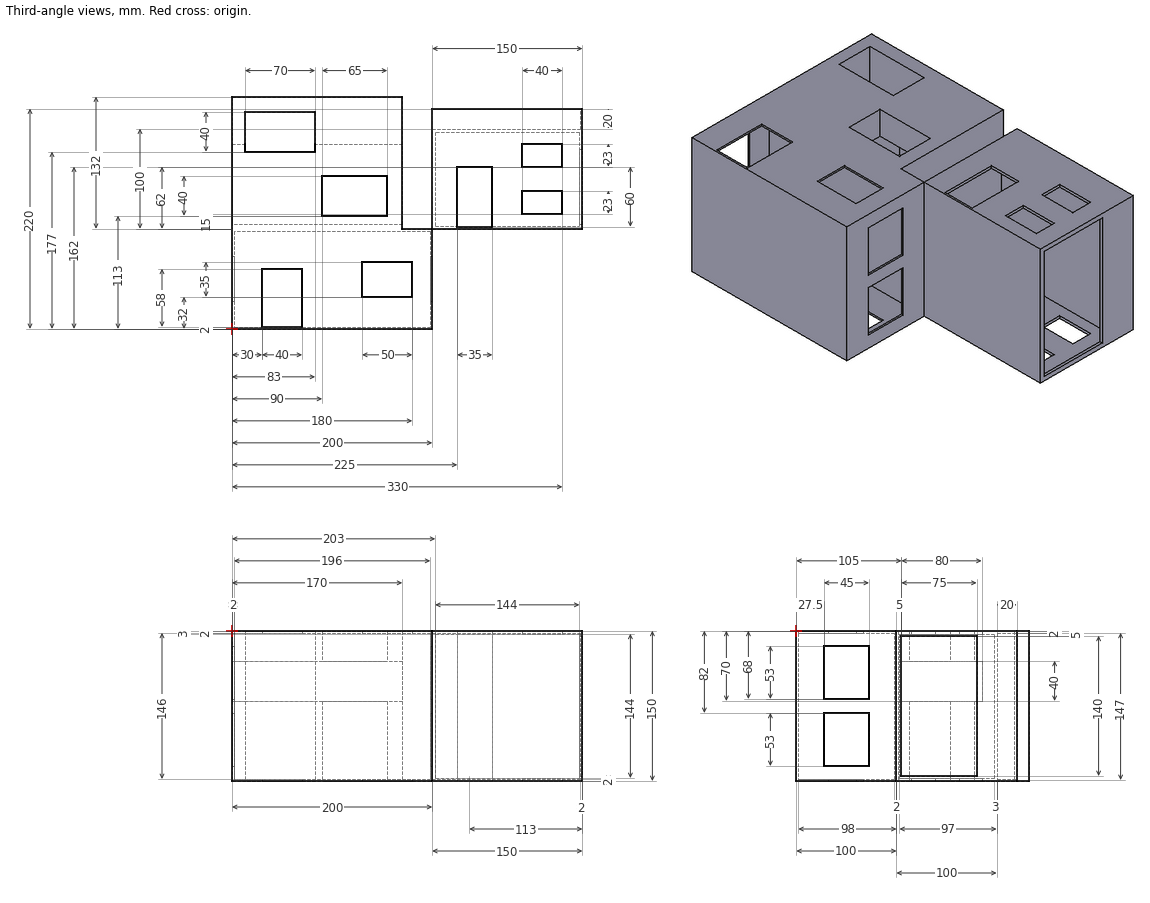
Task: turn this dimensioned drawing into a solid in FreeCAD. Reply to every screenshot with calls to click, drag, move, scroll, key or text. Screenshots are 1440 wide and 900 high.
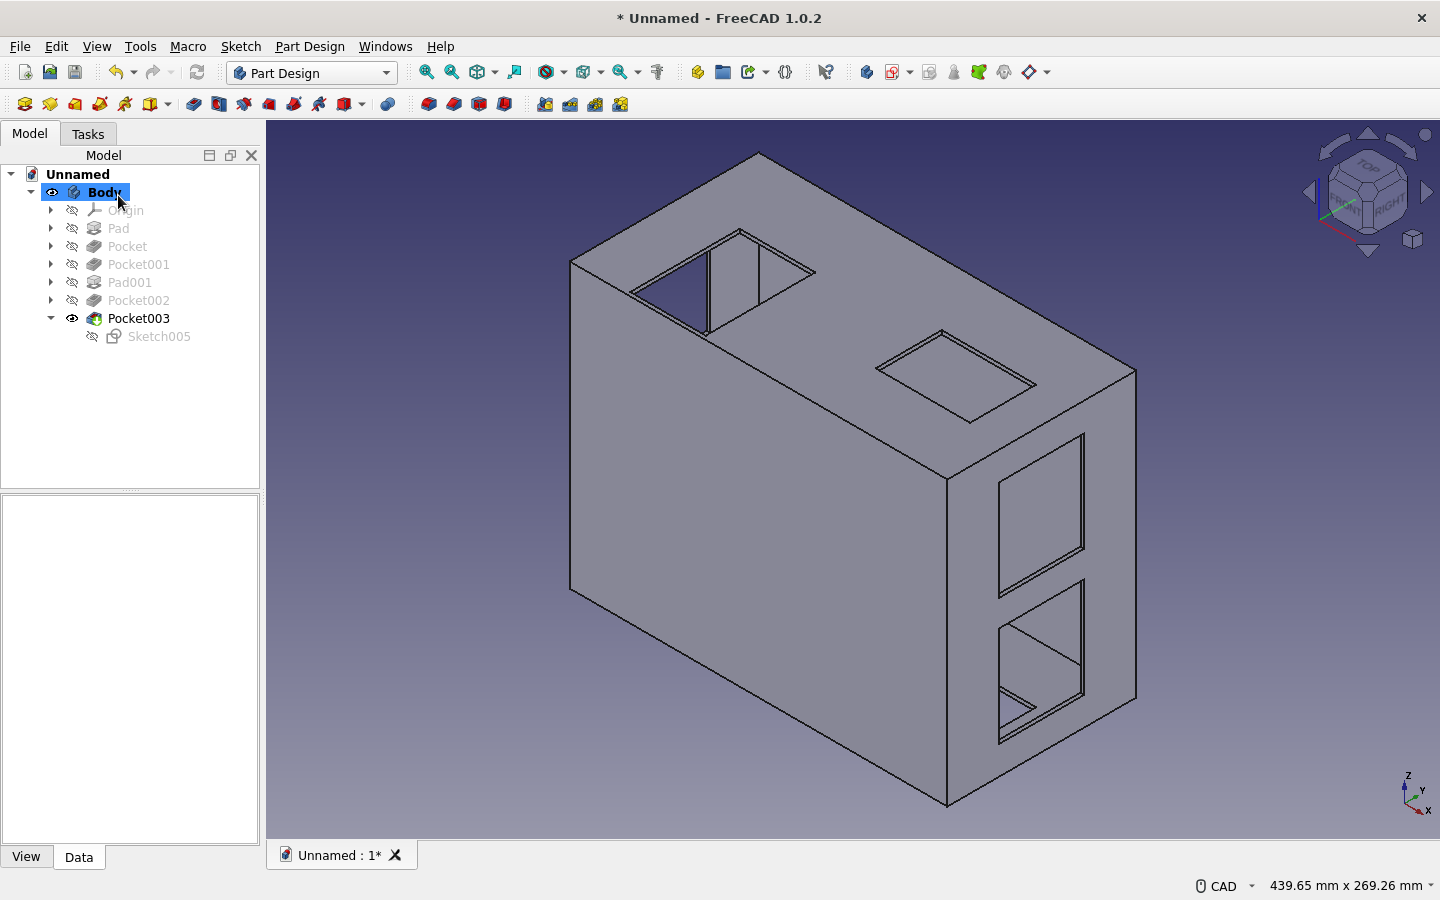
key(4)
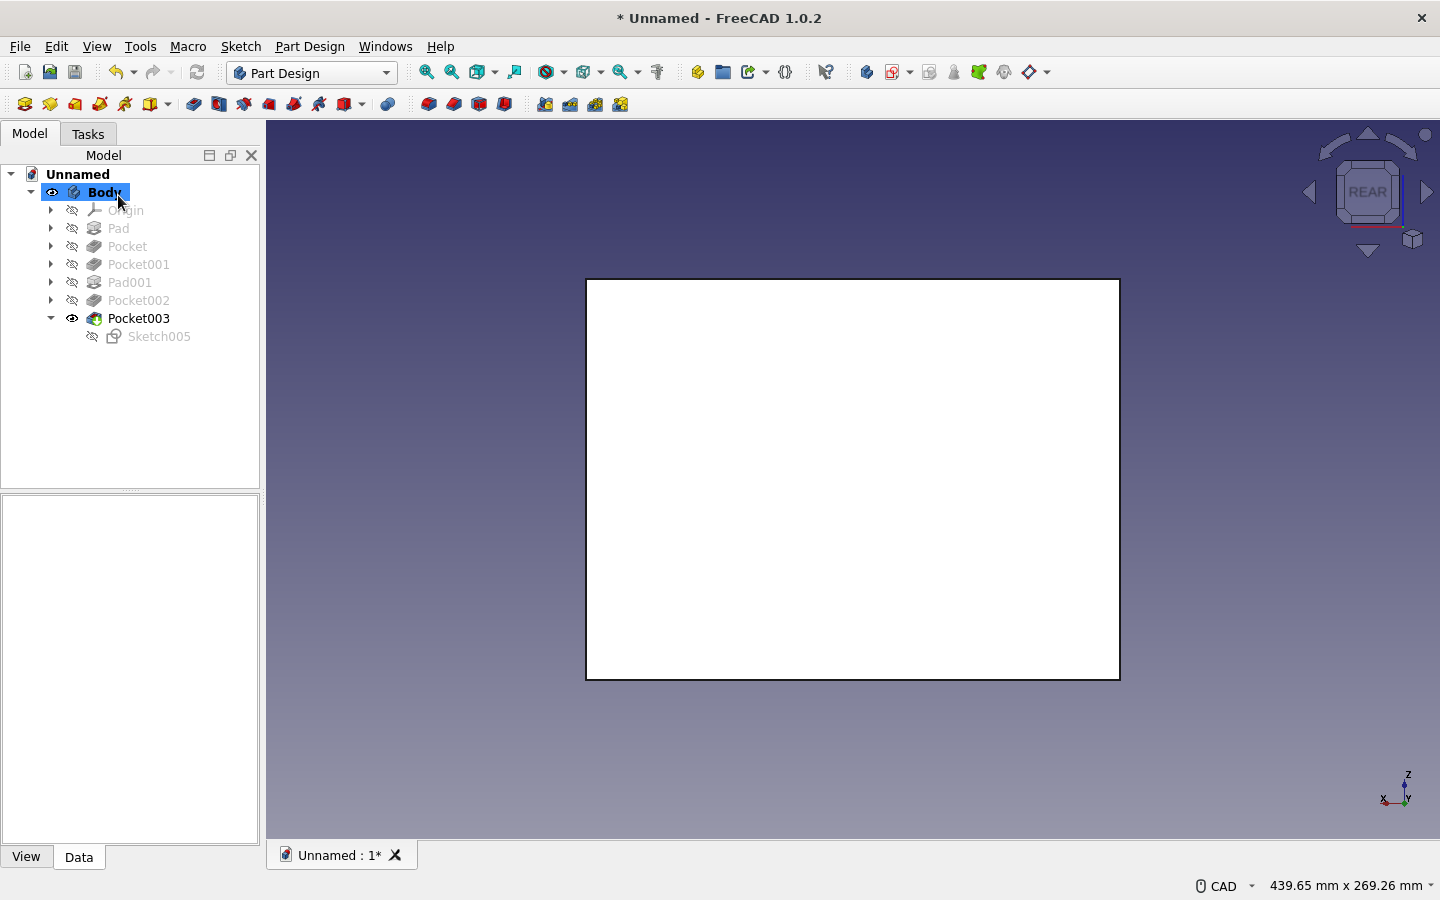
click(853, 478)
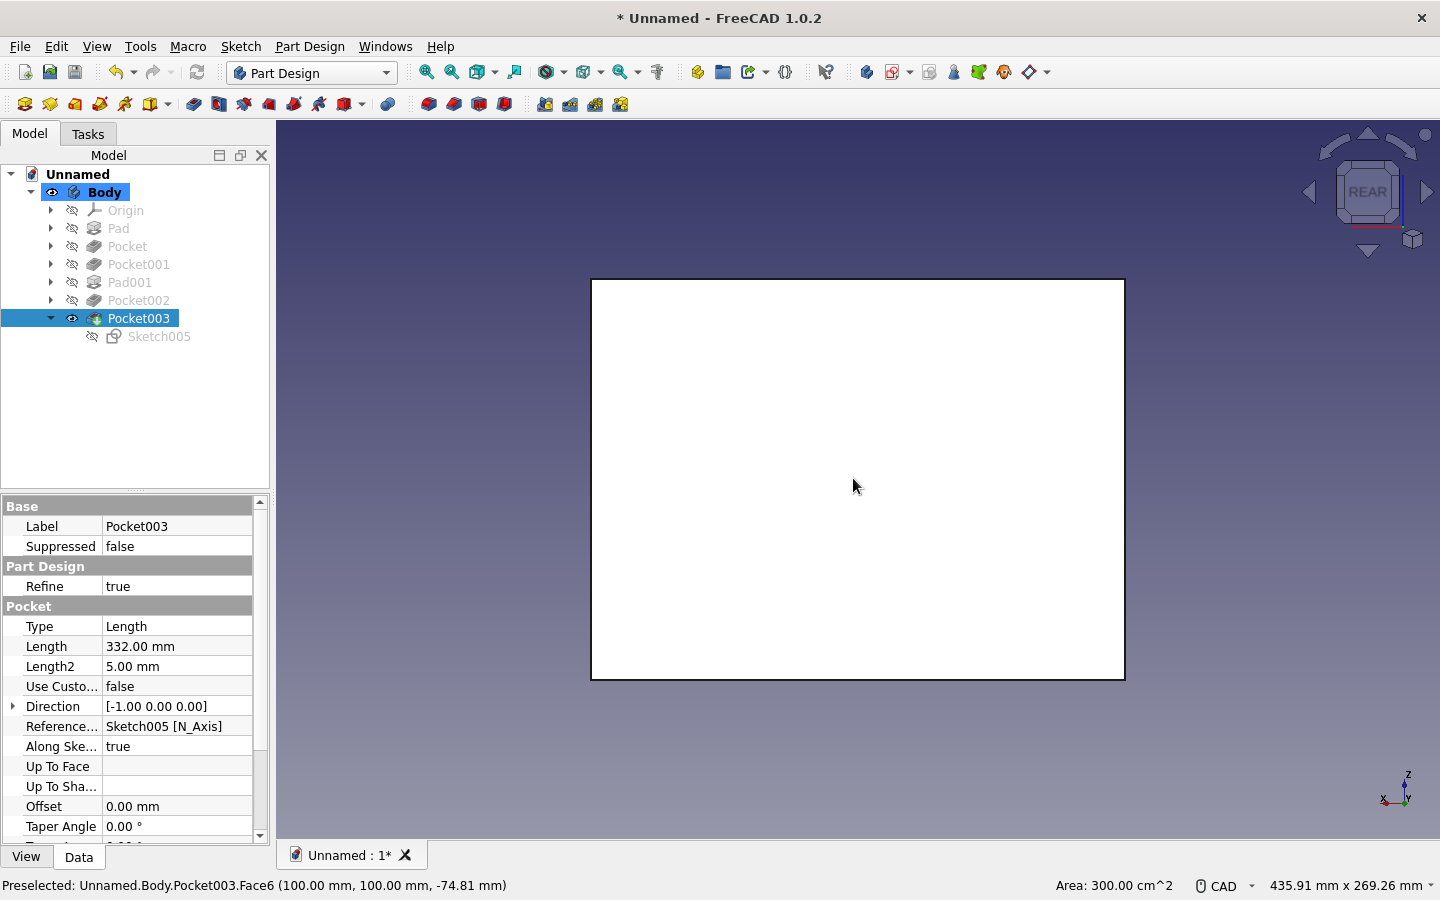
click(892, 72)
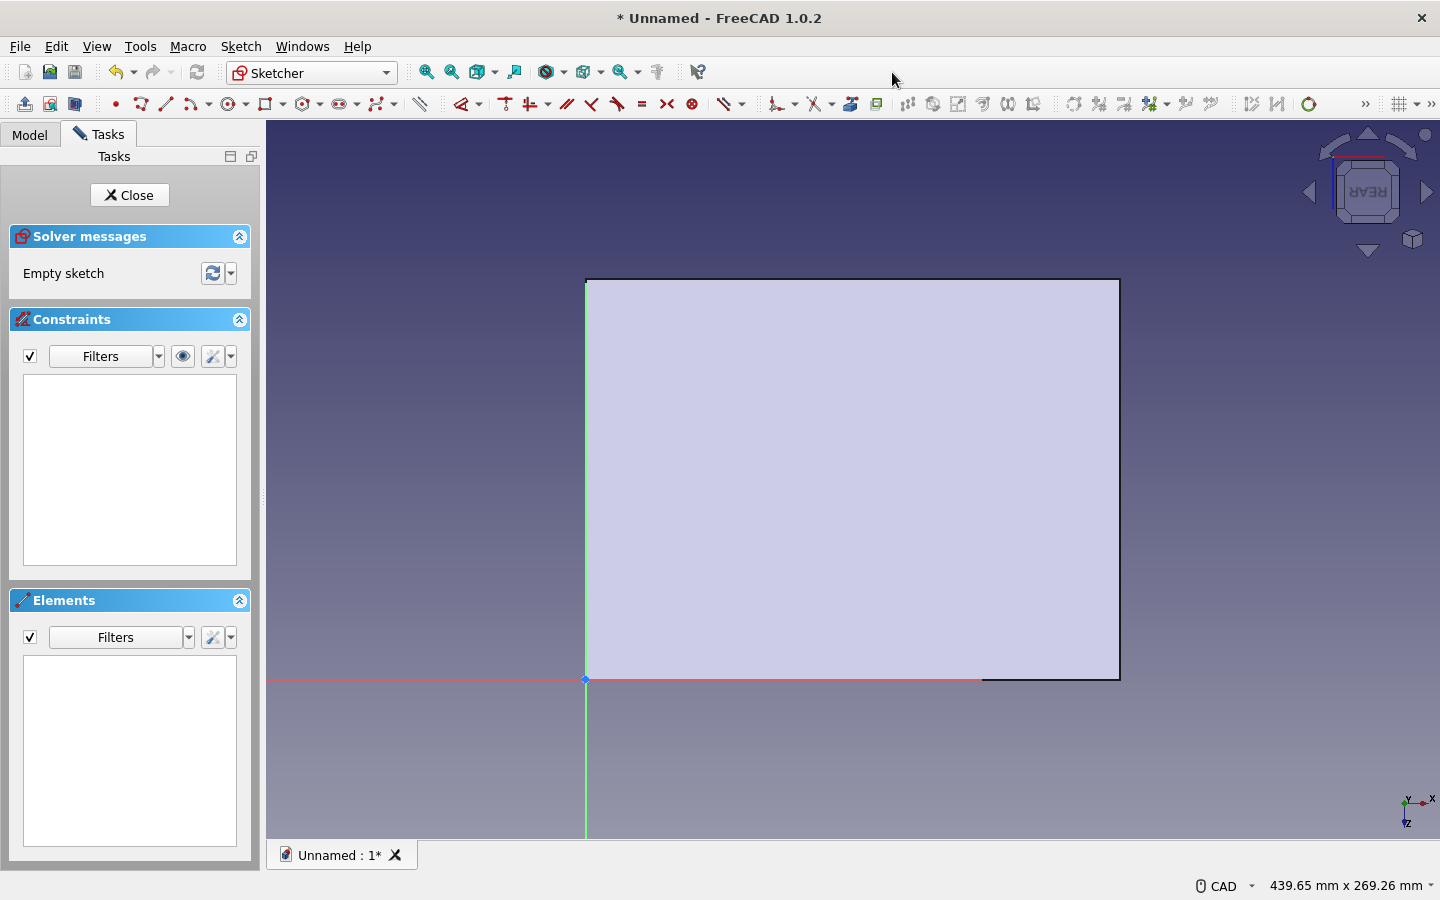
click(264, 104)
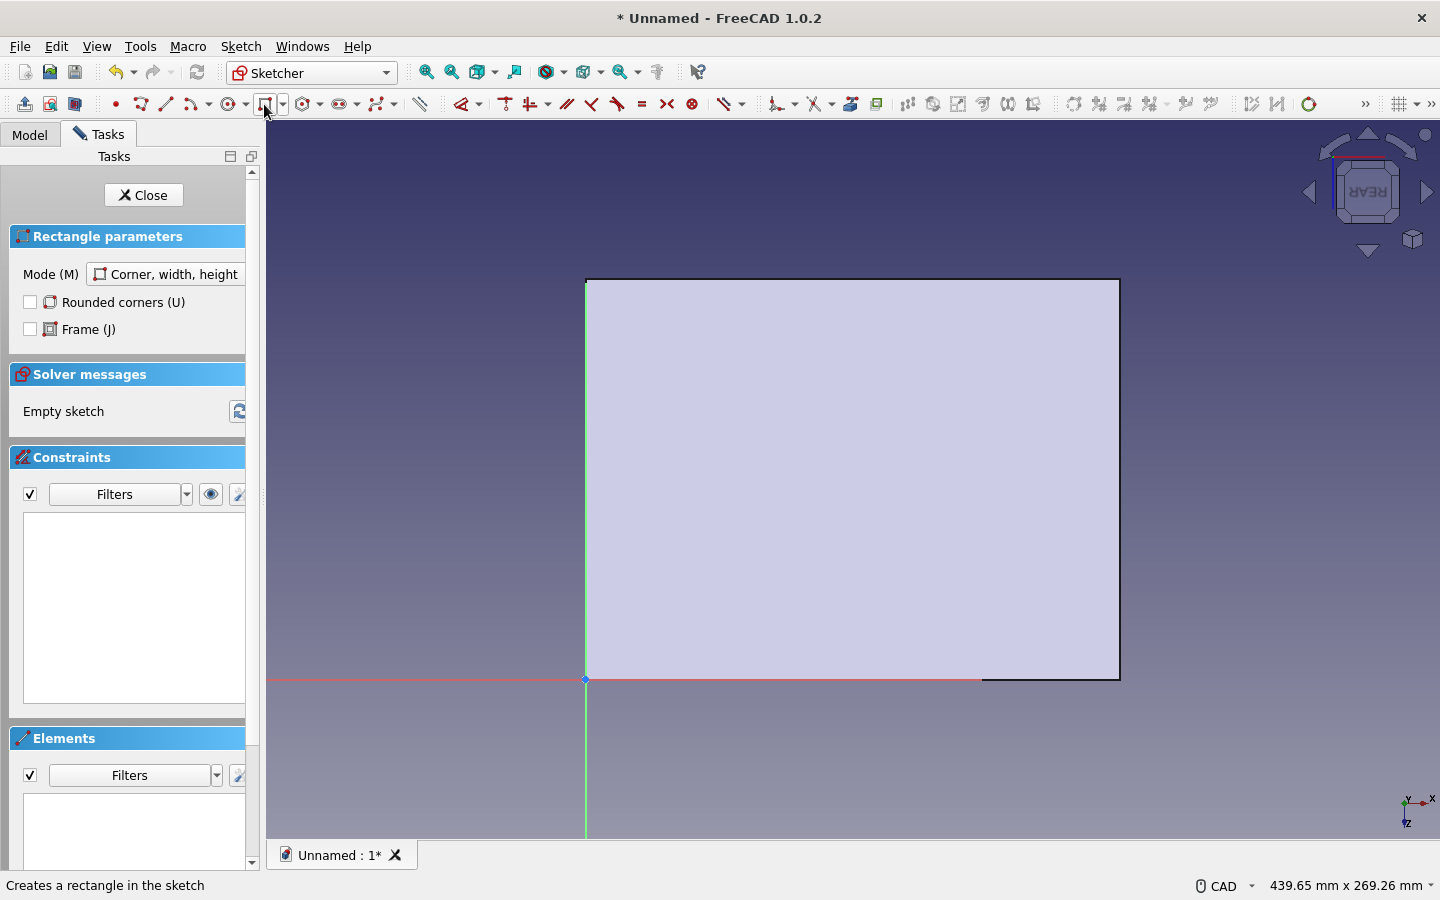
click(586, 680)
move(1040, 279)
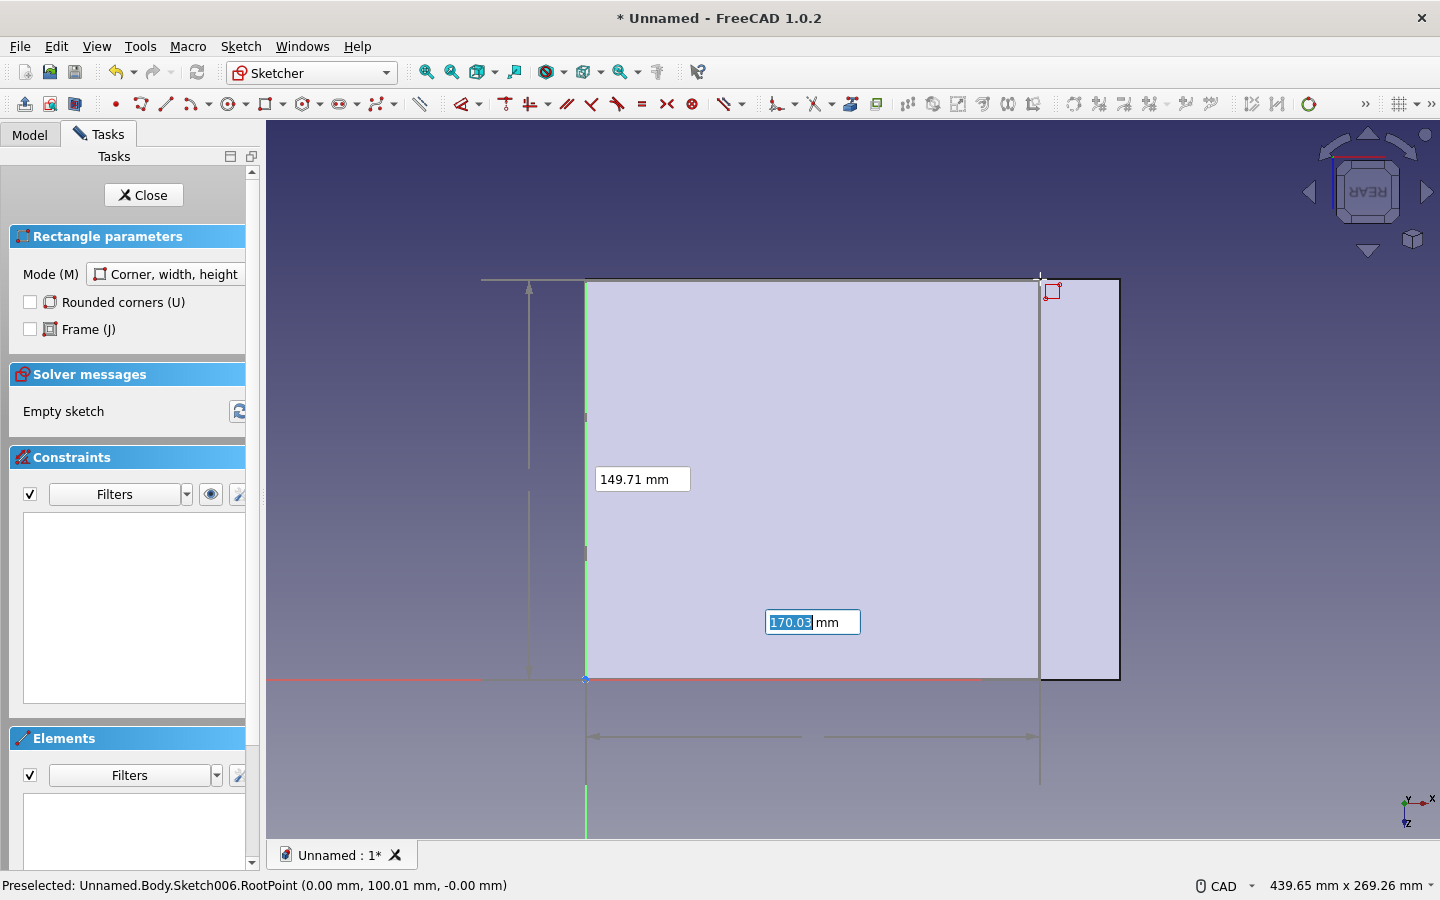
text(170)
key(Tab)
text(150)
key(Return)
key(Escape)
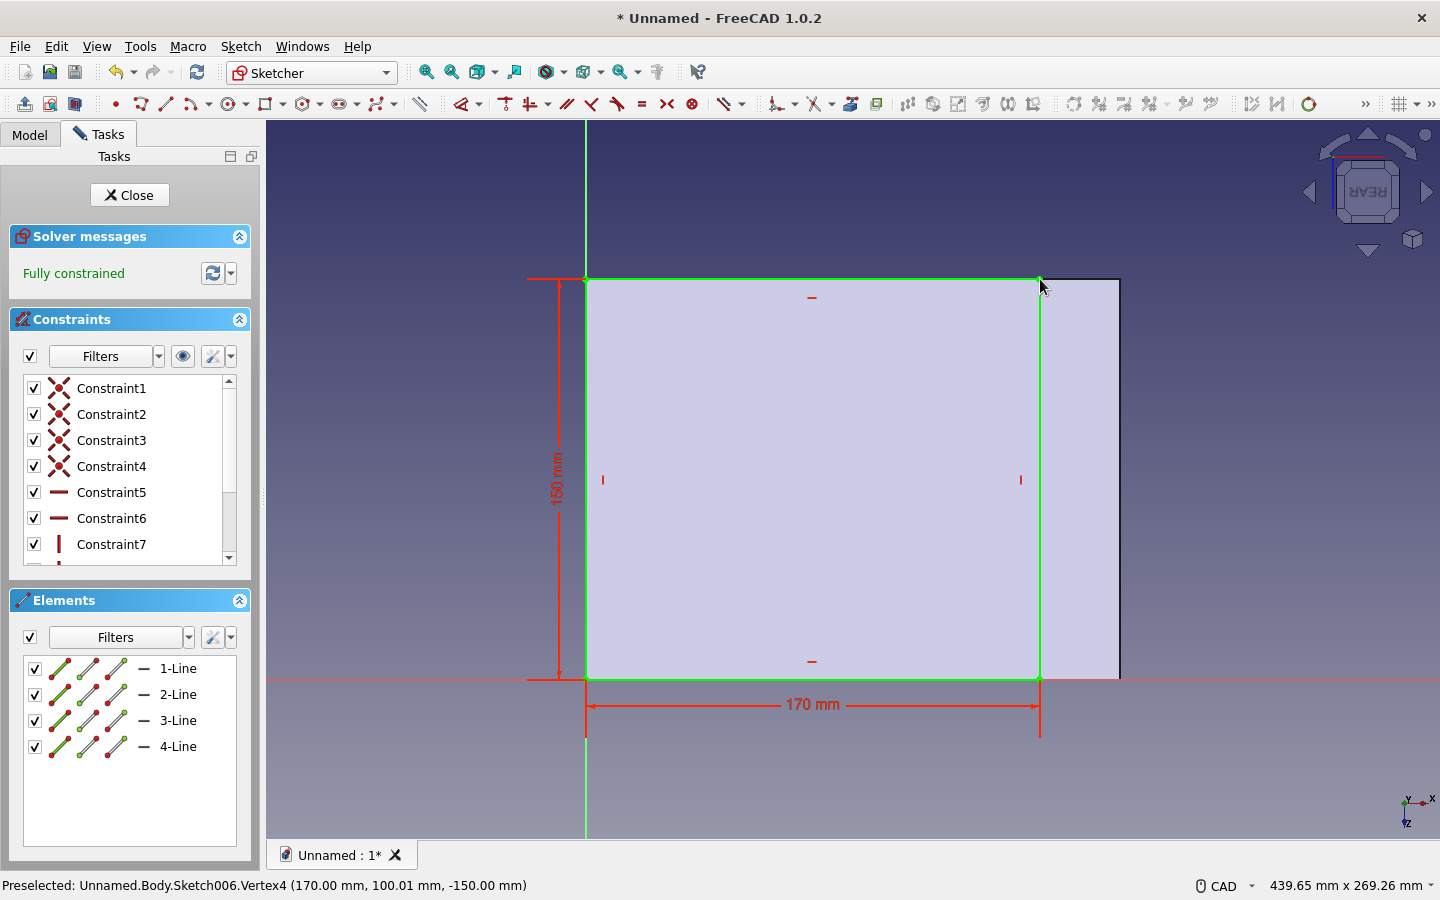
click(130, 195)